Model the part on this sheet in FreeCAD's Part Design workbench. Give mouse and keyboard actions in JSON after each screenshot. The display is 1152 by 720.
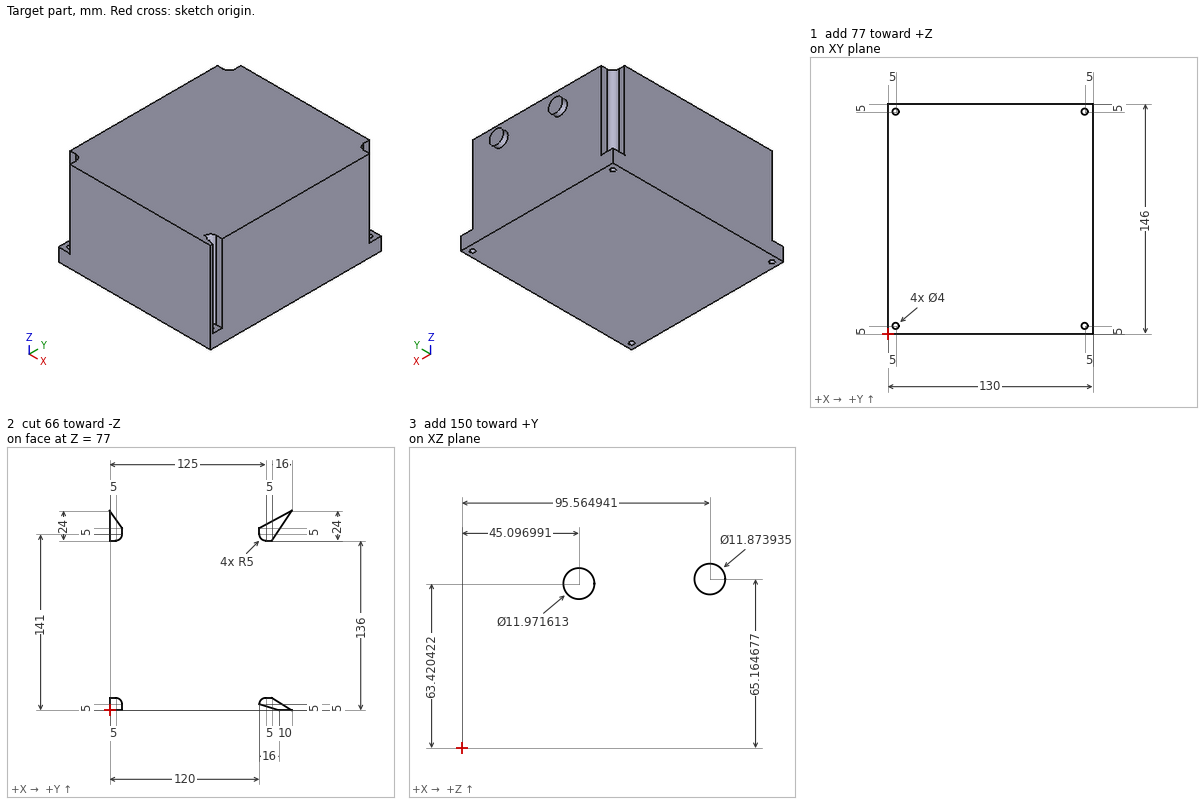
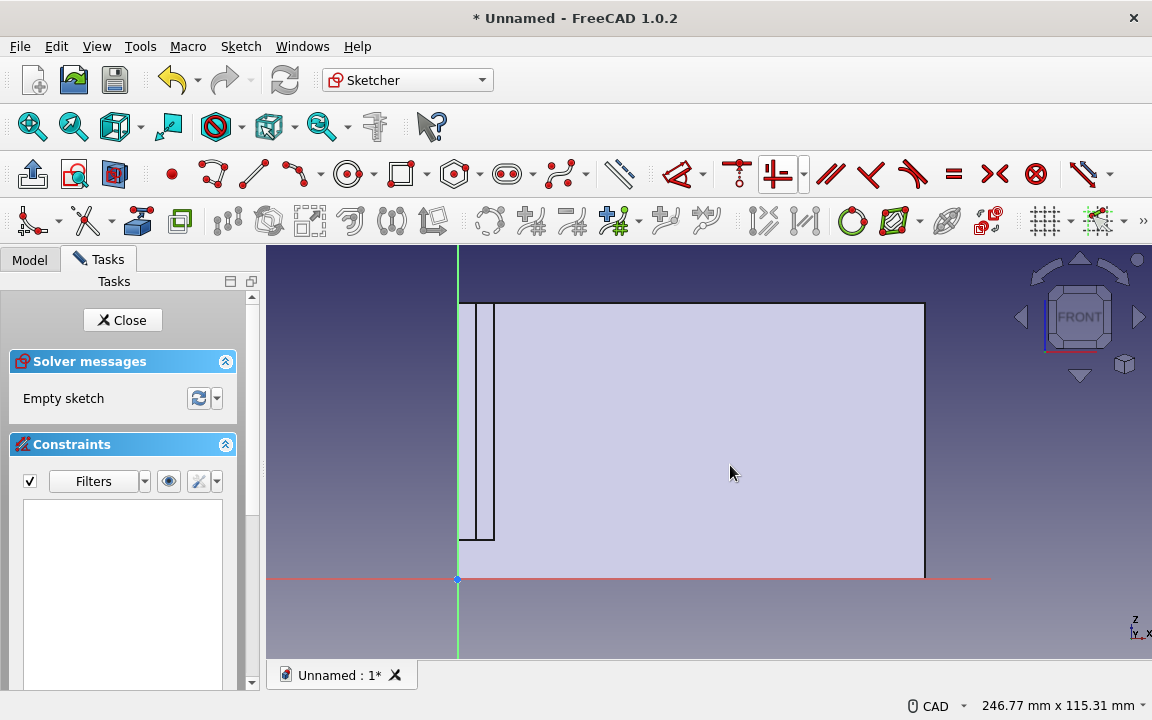
{"action": "left_click", "coordinate": [348, 174]}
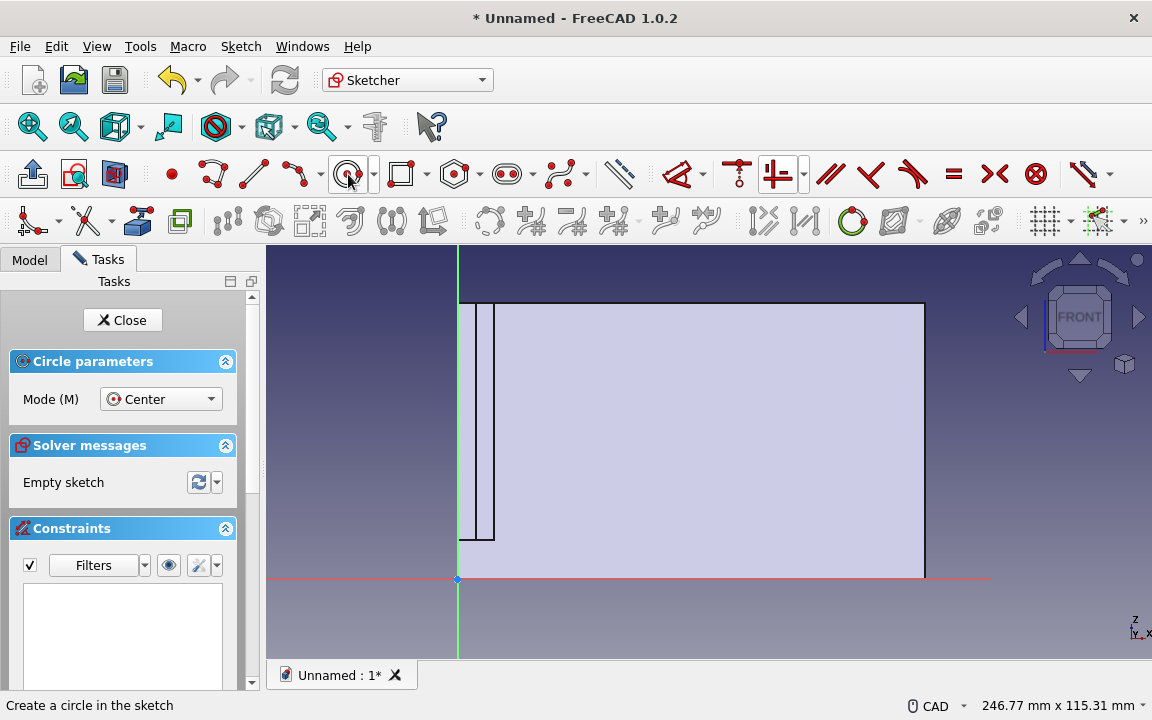
{"action": "left_click", "coordinate": [620, 351]}
{"action": "mouse_move", "coordinate": [635, 336]}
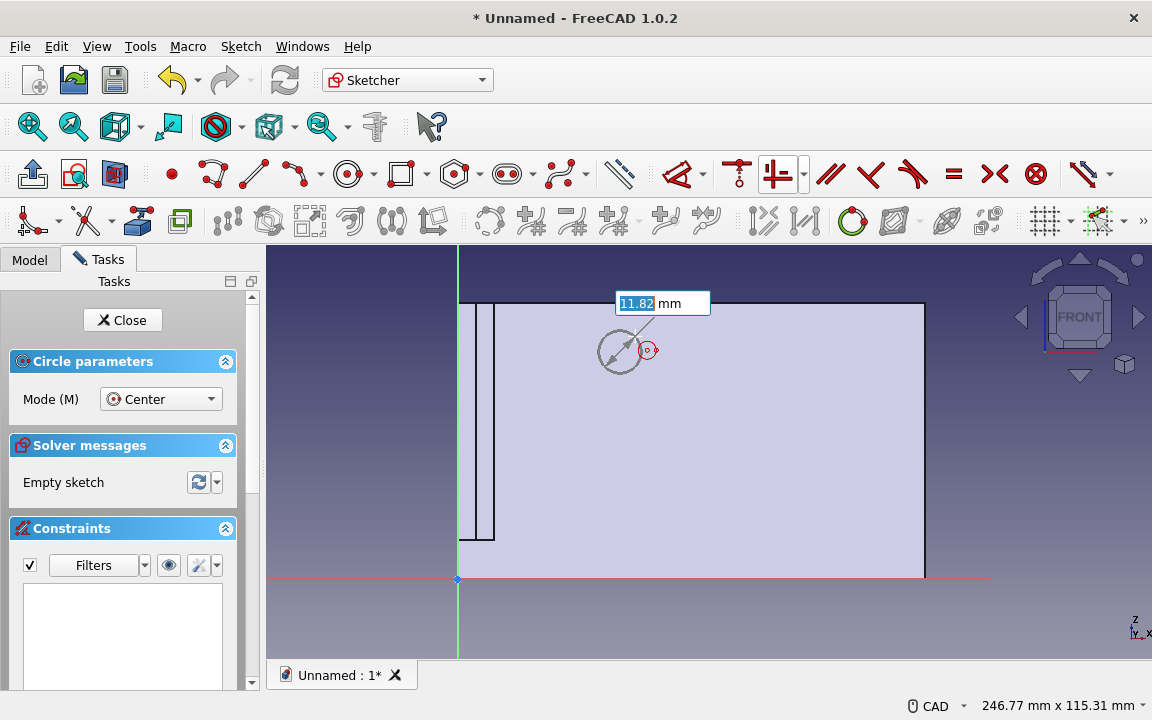
{"action": "type", "text": "11.971613"}
{"action": "key", "text": "Return"}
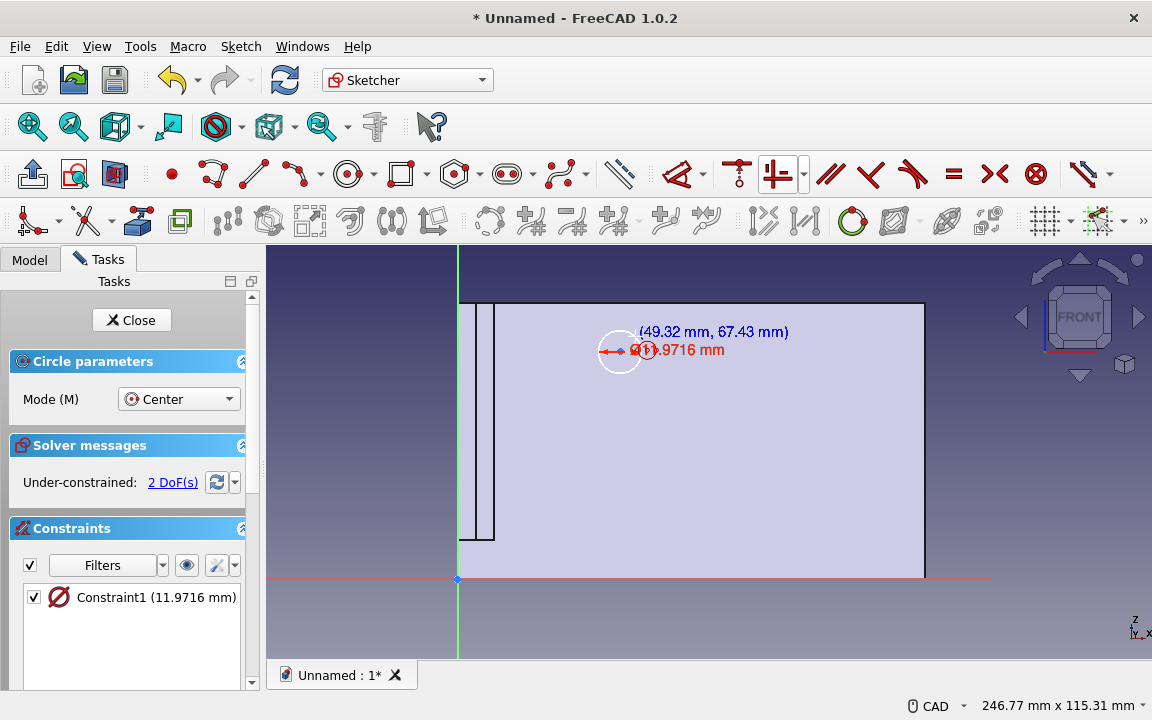
{"action": "left_click", "coordinate": [801, 345]}
{"action": "mouse_move", "coordinate": [816, 330]}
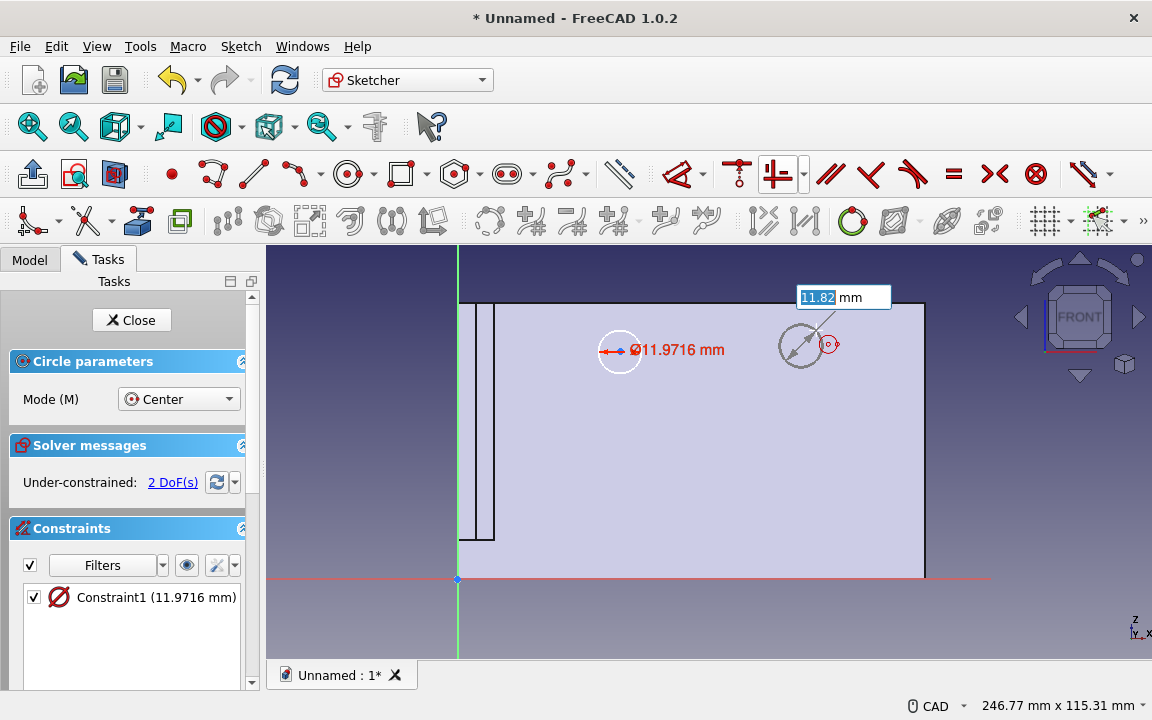
{"action": "type", "text": "11.873935"}
{"action": "key", "text": "Return"}
{"action": "key", "text": "Escape"}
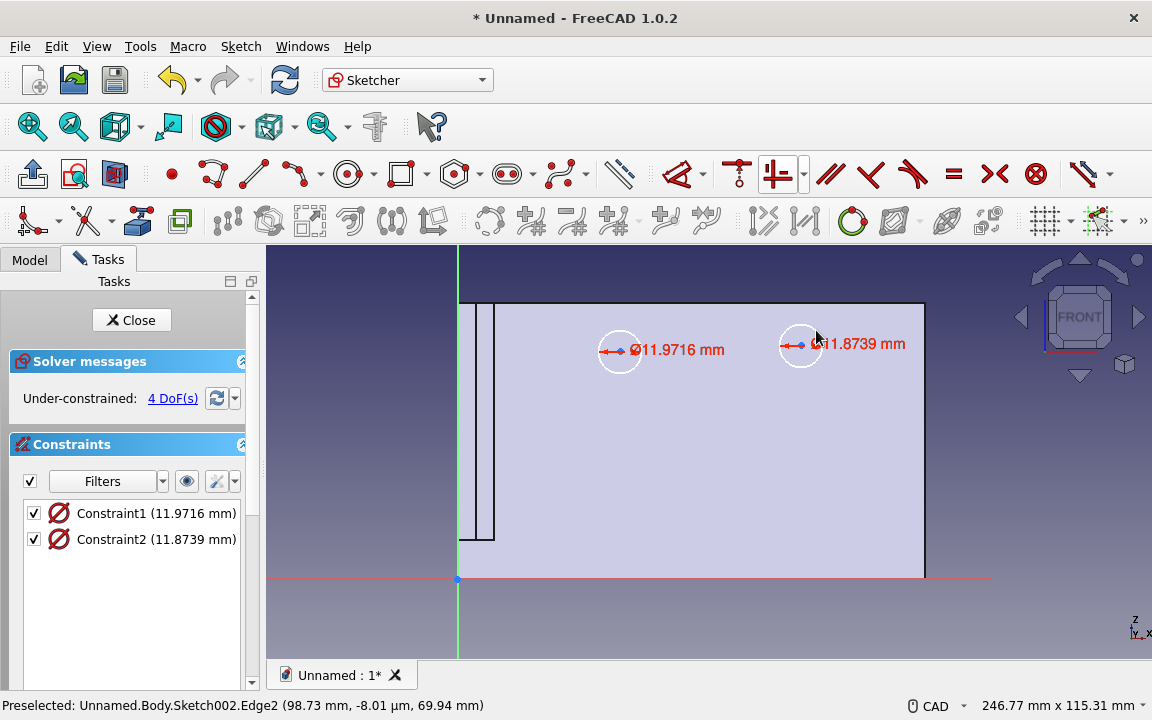
{"action": "left_click", "coordinate": [676, 174]}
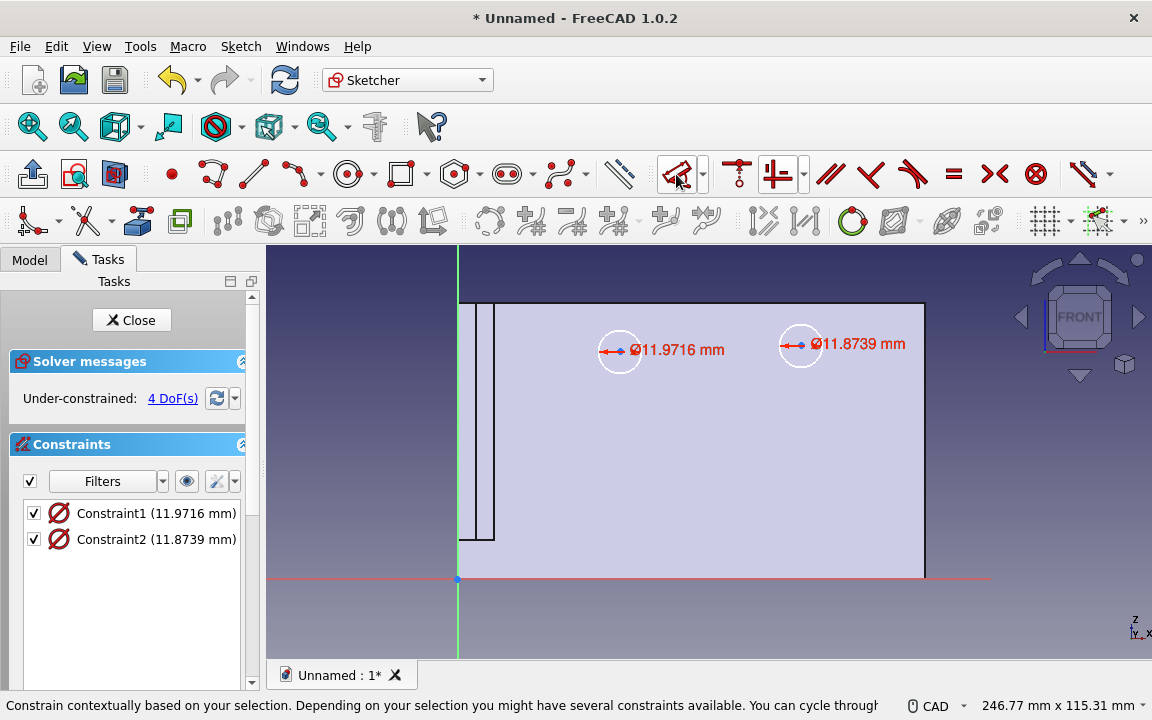
{"action": "left_click", "coordinate": [620, 352]}
{"action": "left_click", "coordinate": [539, 613]}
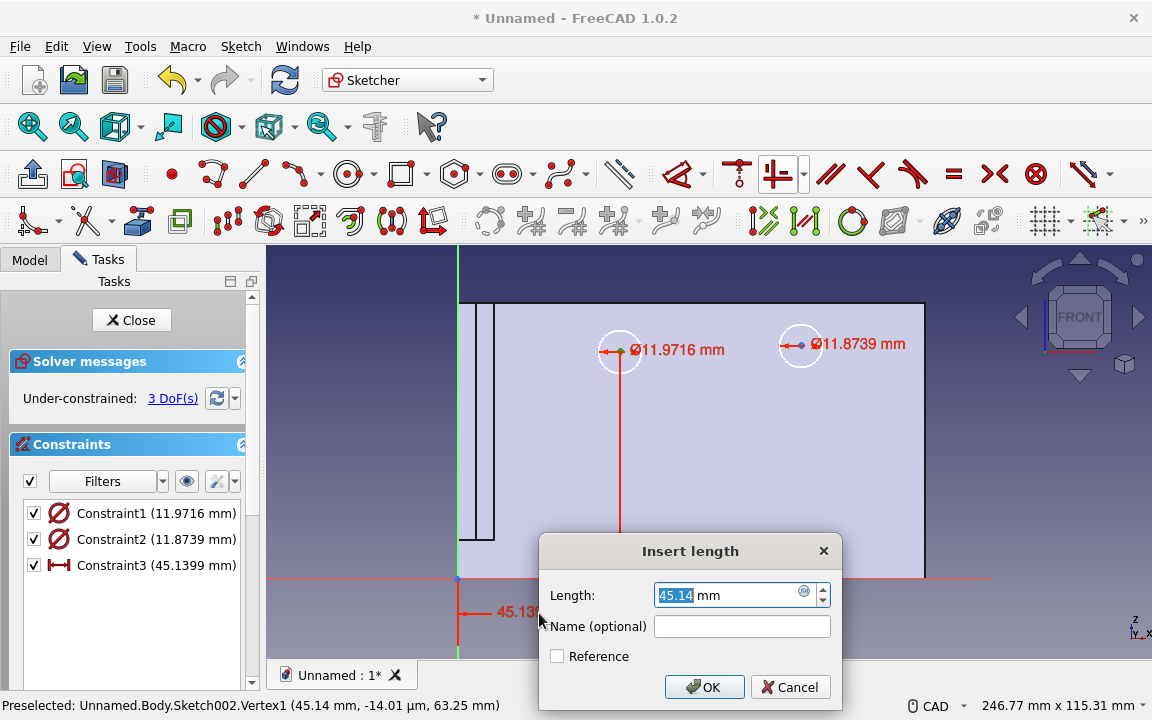
{"action": "type", "text": "45.096991"}
{"action": "key", "text": "Return"}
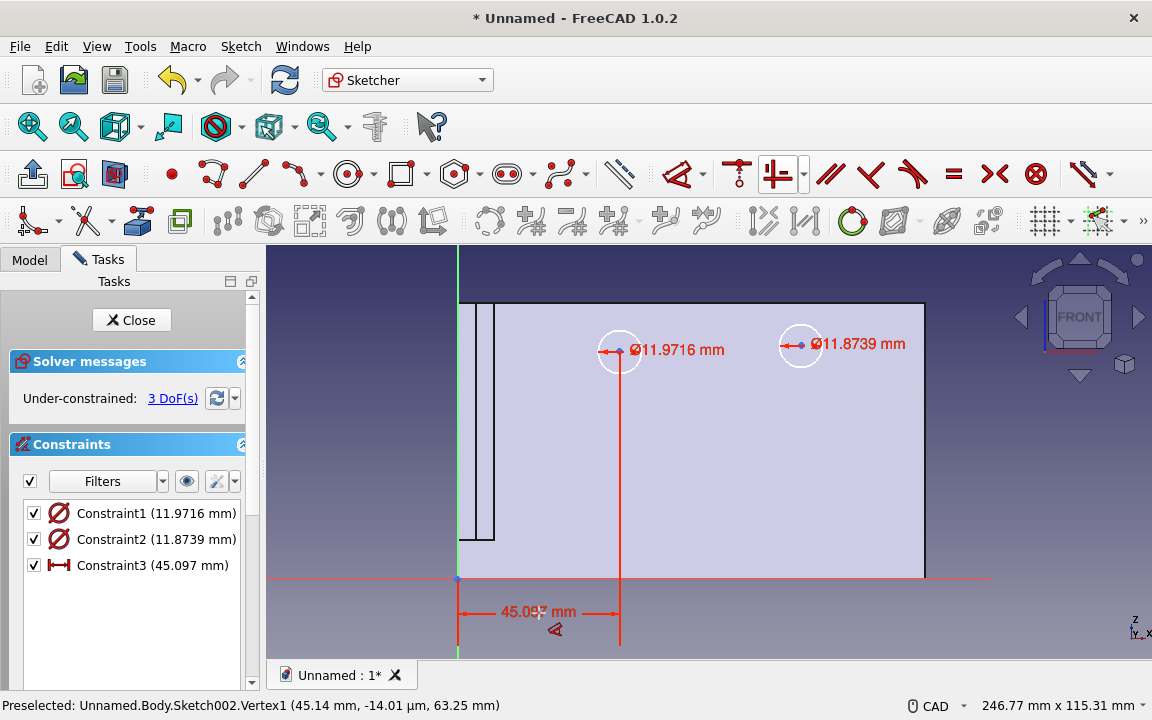
{"action": "left_click", "coordinate": [620, 352]}
{"action": "left_click", "coordinate": [424, 466]}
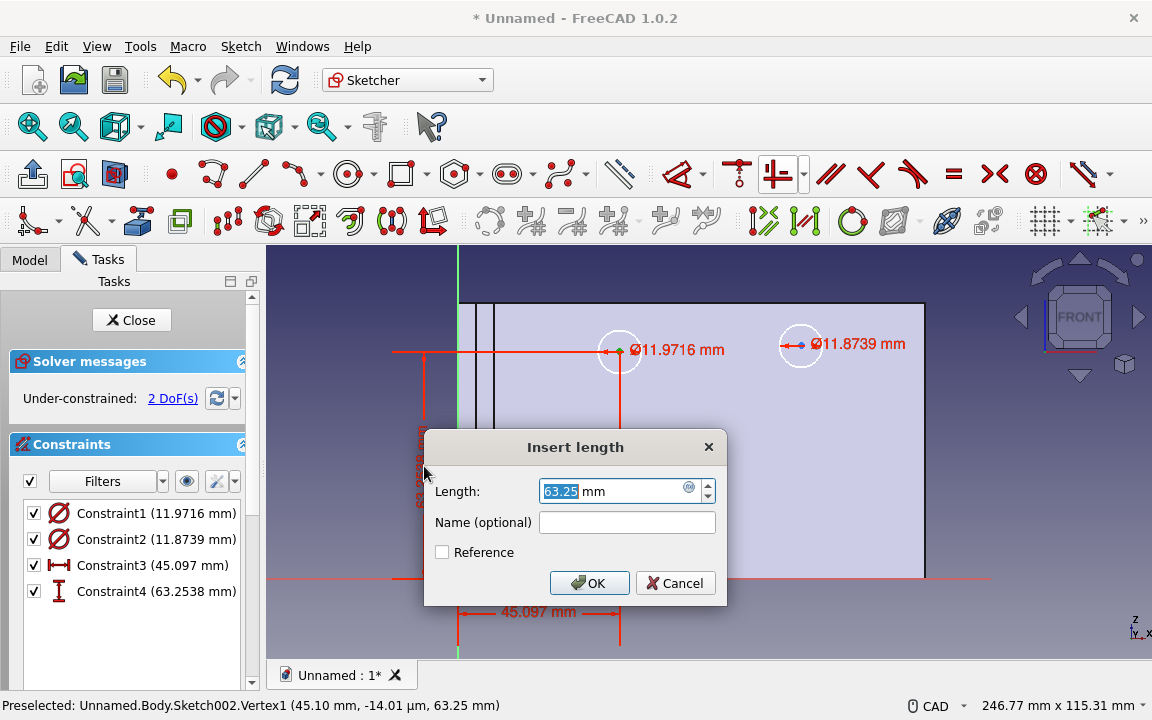
{"action": "type", "text": "63.420422"}
{"action": "key", "text": "Return"}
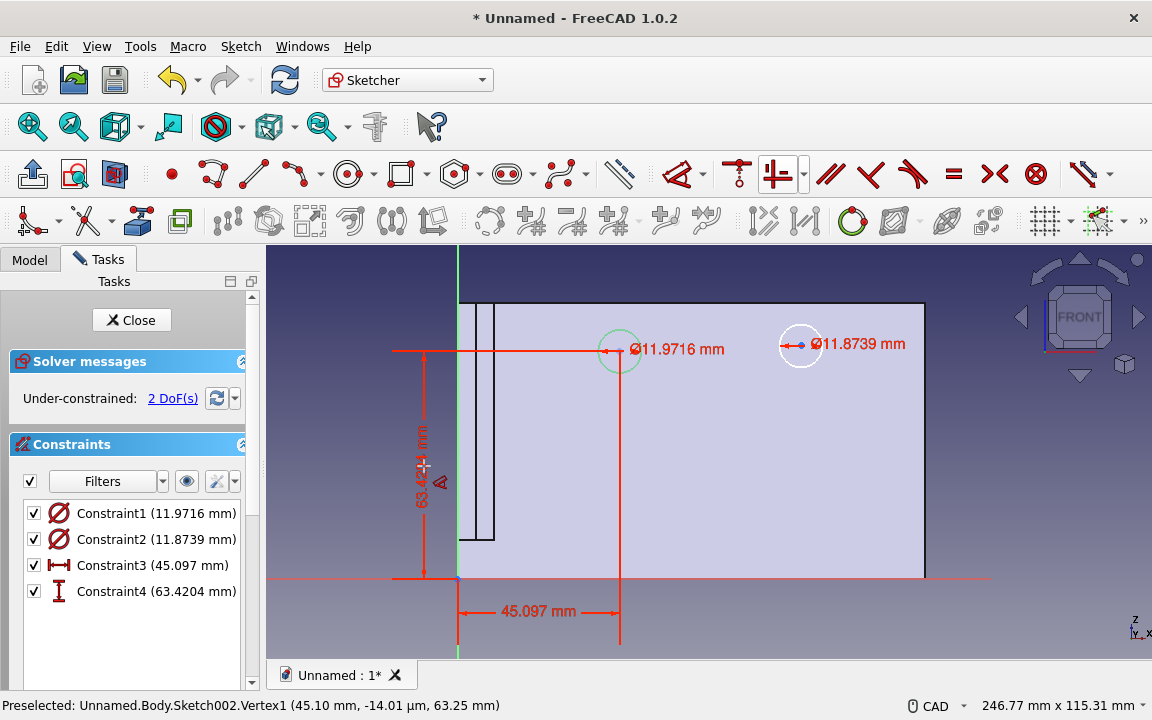
{"action": "left_click", "coordinate": [801, 346]}
{"action": "left_click", "coordinate": [629, 613]}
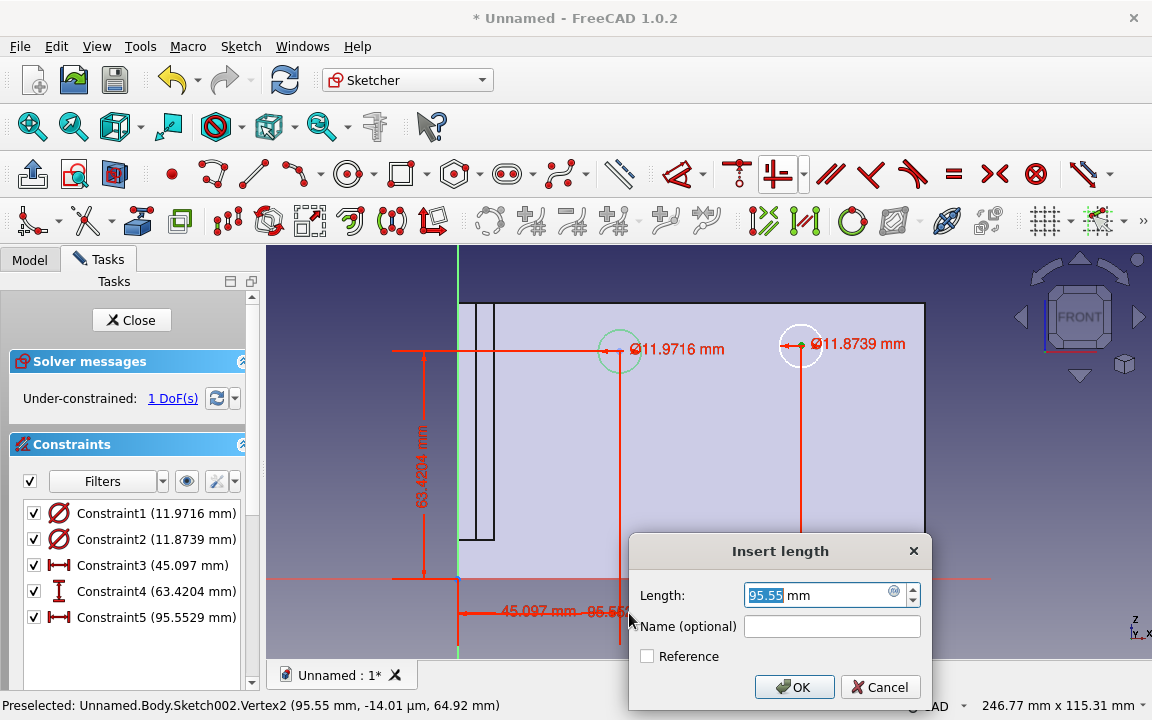
{"action": "type", "text": "95.564941"}
{"action": "key", "text": "Return"}